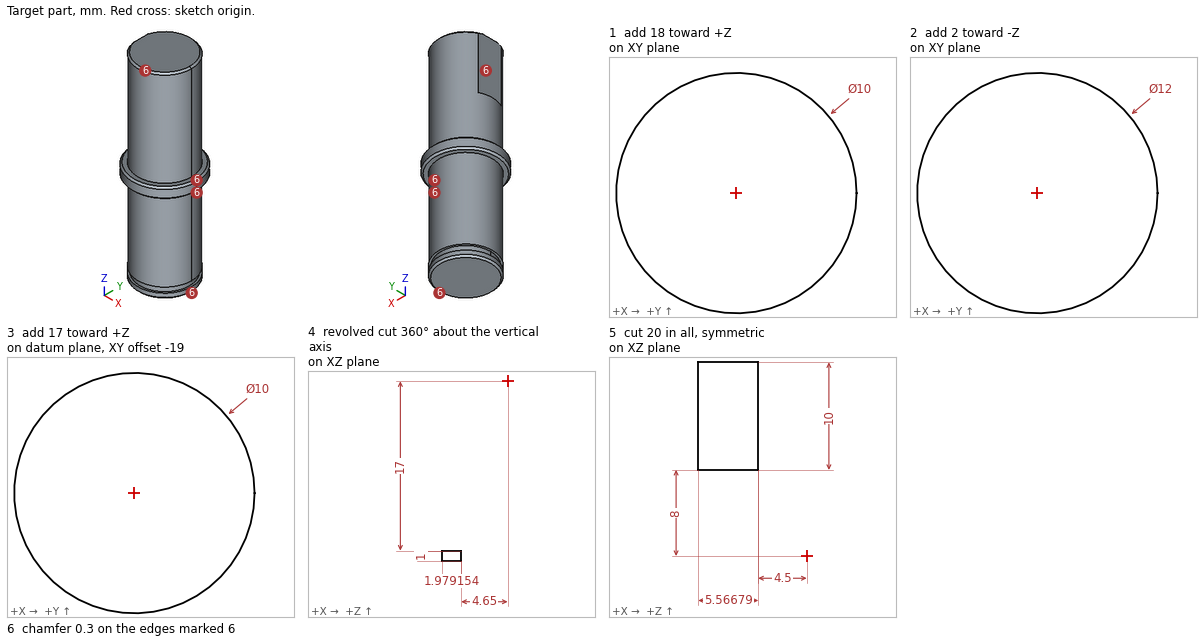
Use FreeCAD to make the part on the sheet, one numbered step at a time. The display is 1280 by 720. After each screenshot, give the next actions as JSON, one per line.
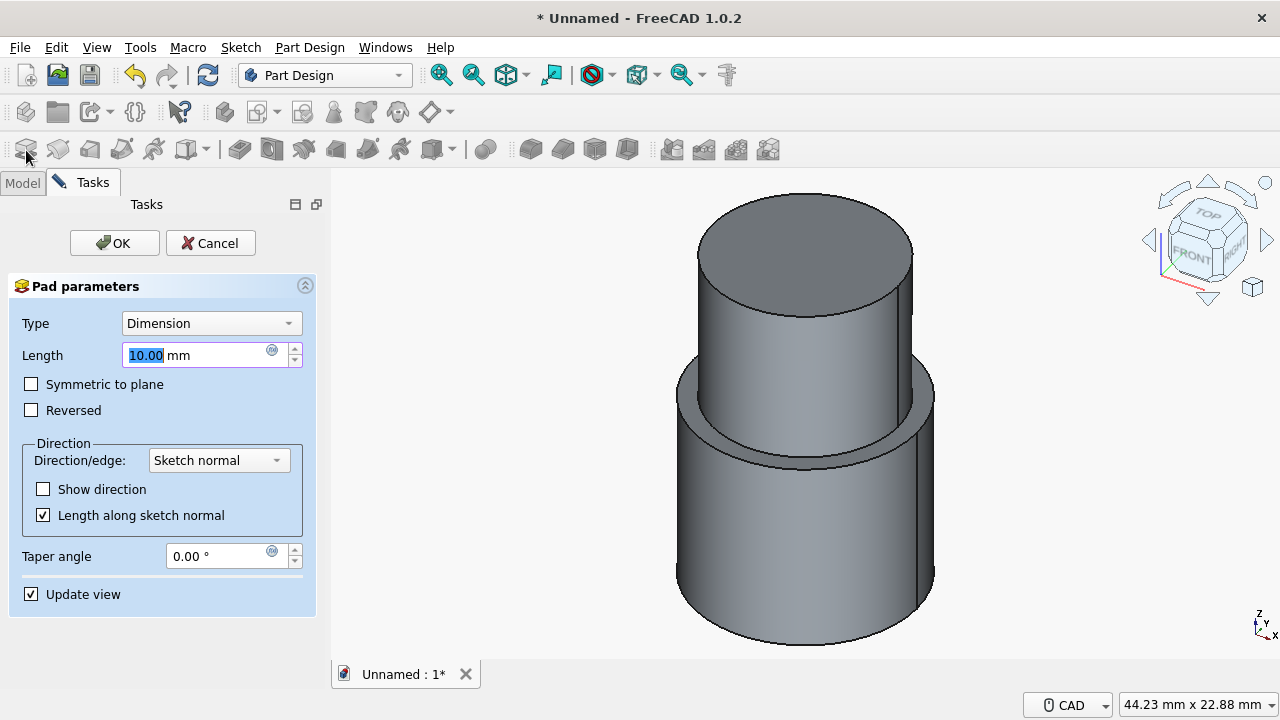
{"action": "type", "text": "2"}
{"action": "key", "text": "Tab"}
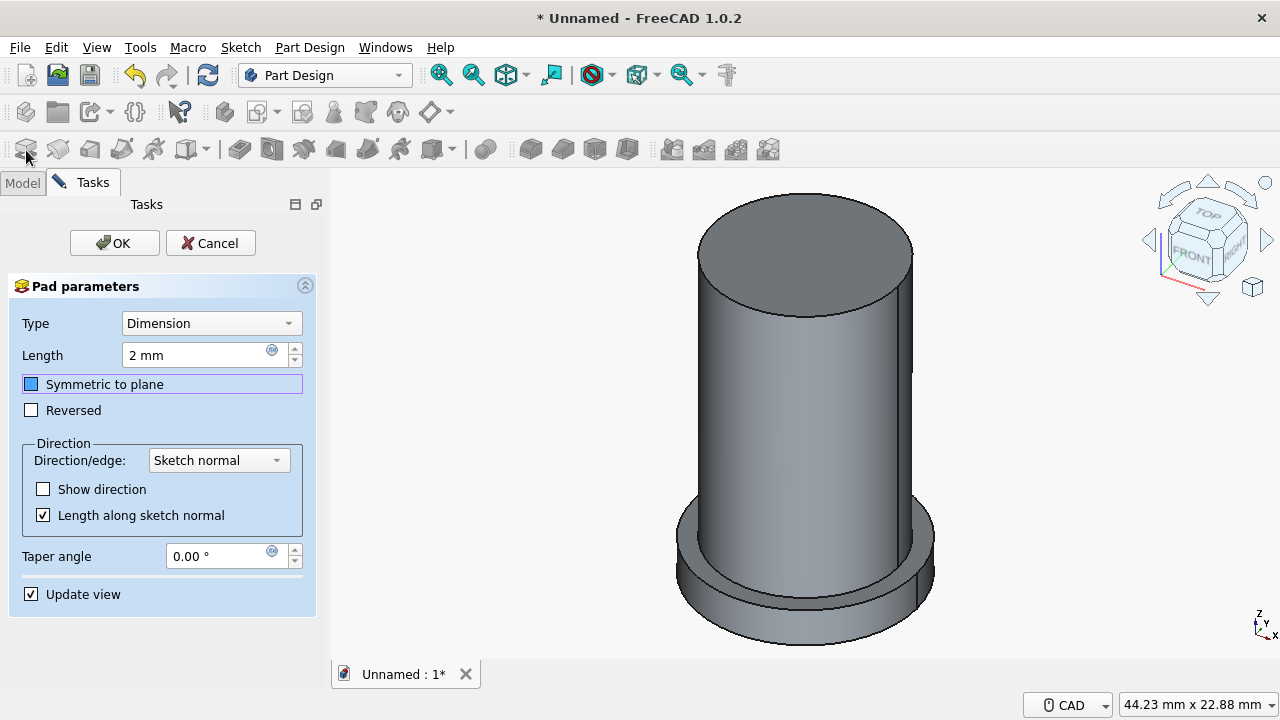
{"action": "left_click", "coordinate": [30, 410]}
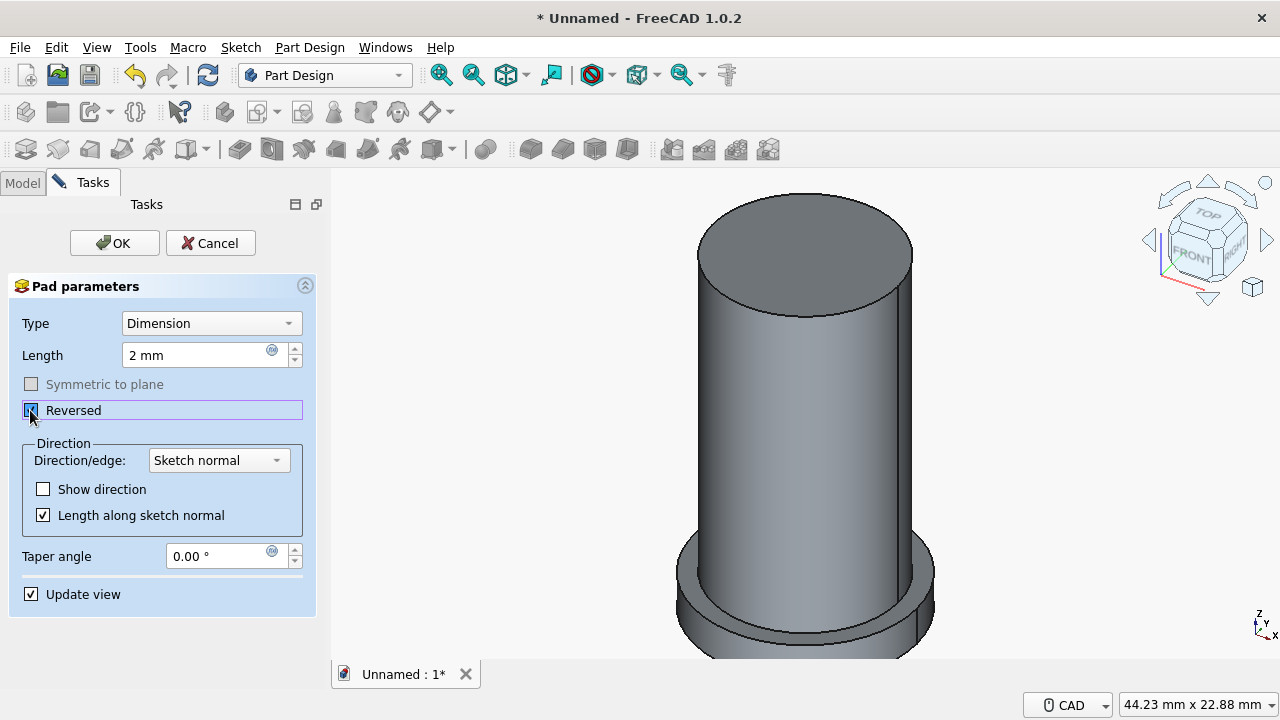
{"action": "left_click", "coordinate": [115, 243]}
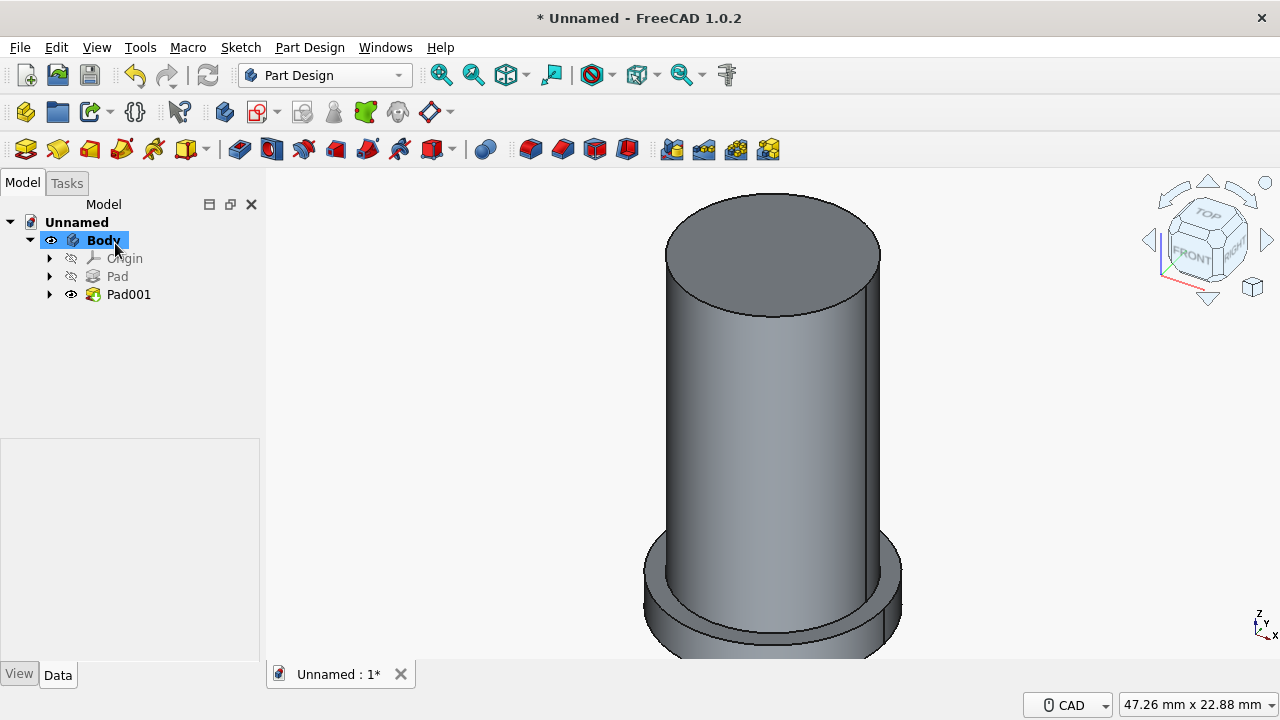
{"action": "left_click", "coordinate": [442, 76]}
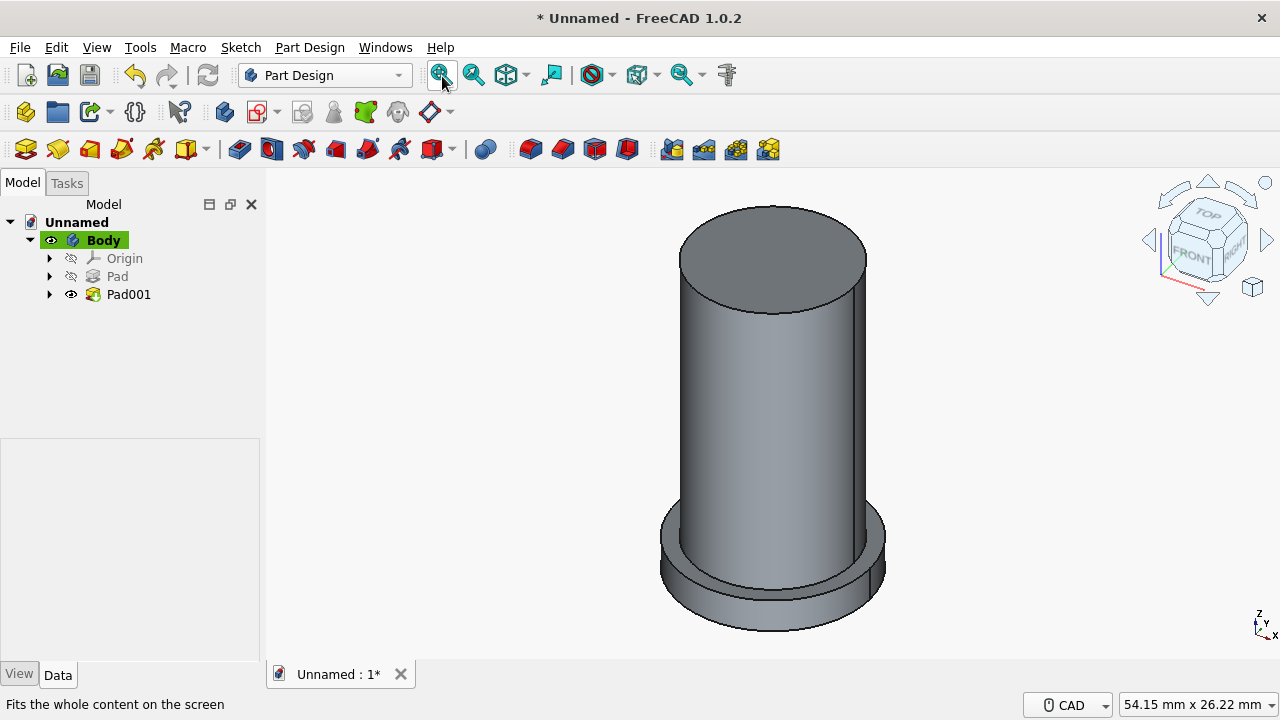
{"action": "left_click", "coordinate": [50, 258]}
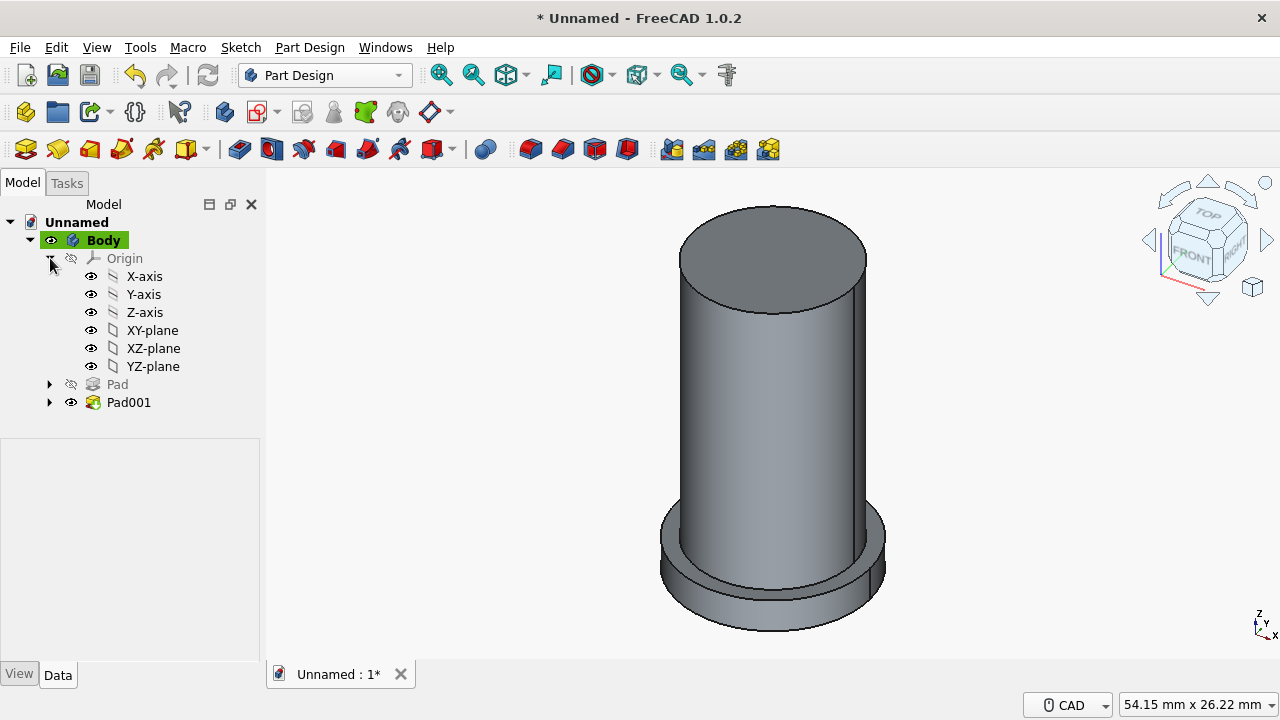
{"action": "left_click", "coordinate": [136, 330]}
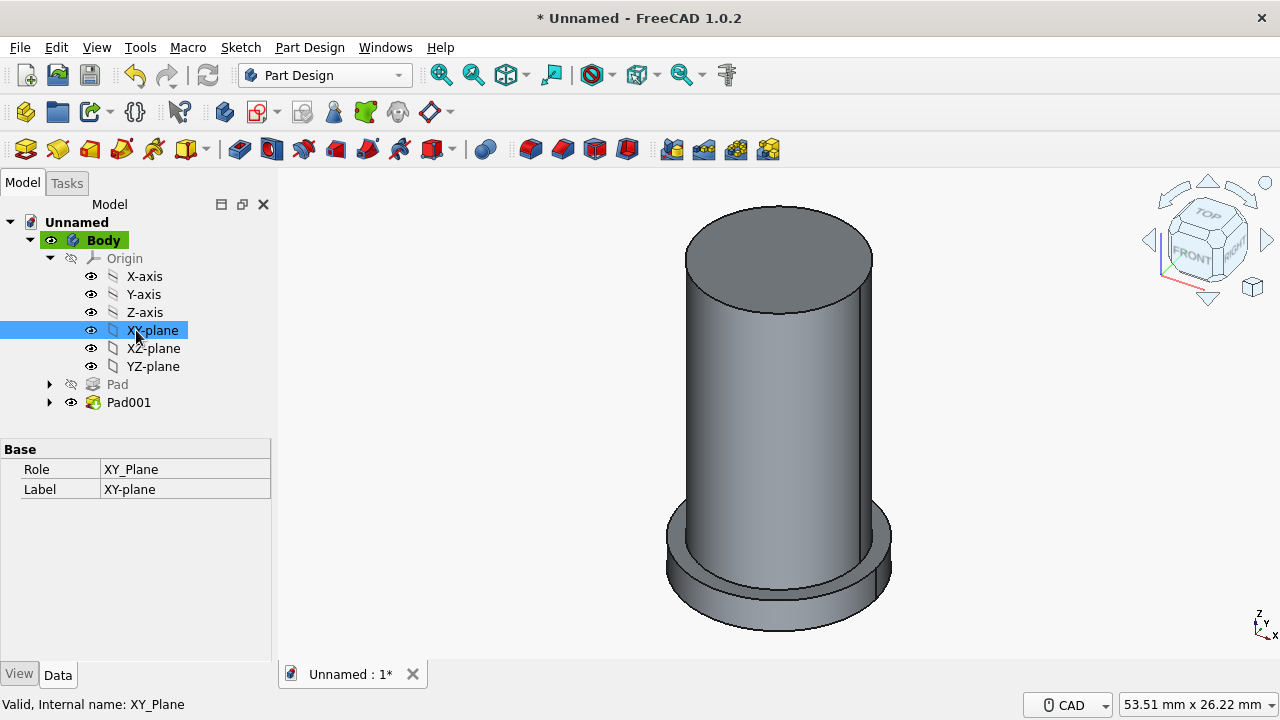
{"action": "left_click", "coordinate": [430, 112]}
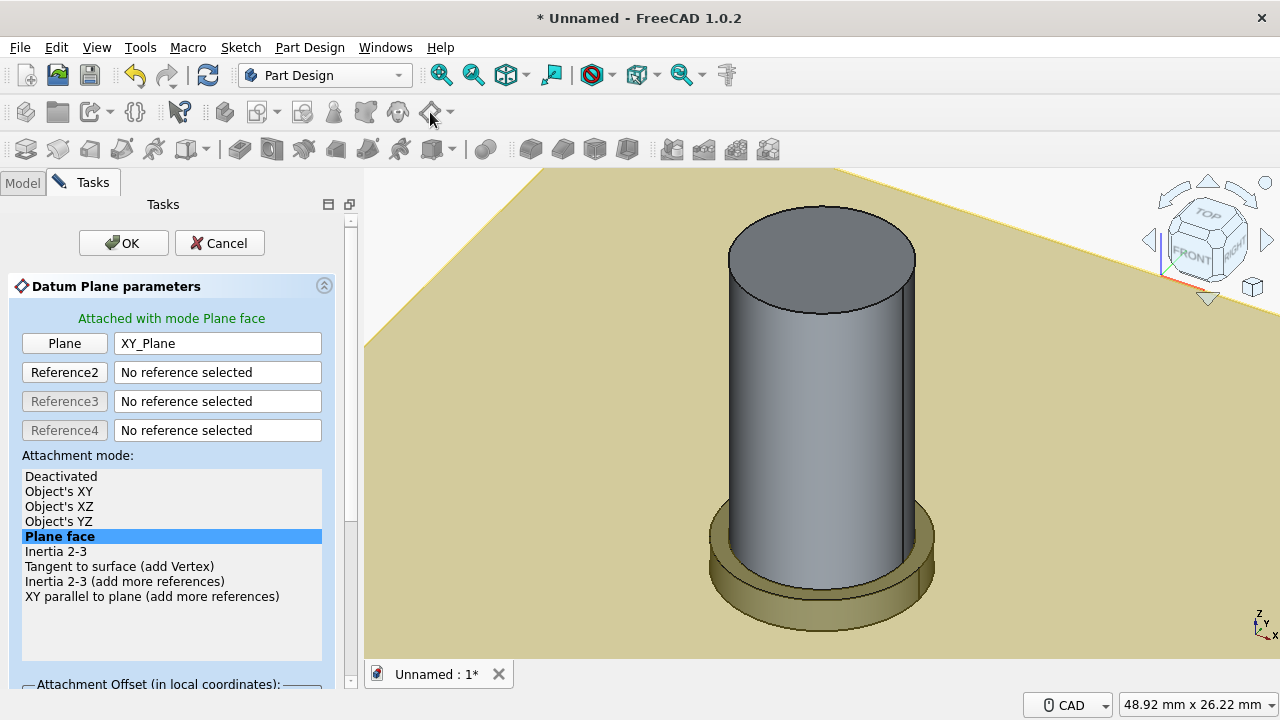
{"action": "scroll", "coordinate": [351, 451], "scroll_direction": "down", "scroll_amount": 3}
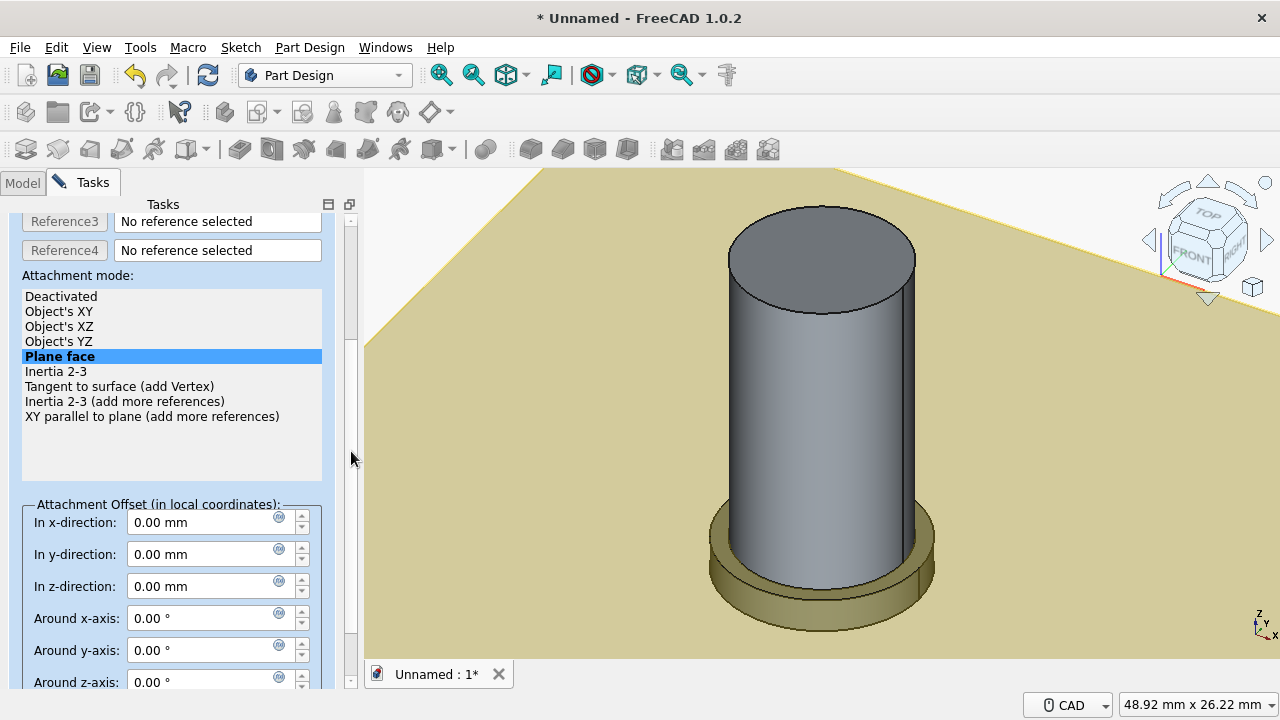
{"action": "triple_click", "coordinate": [210, 586]}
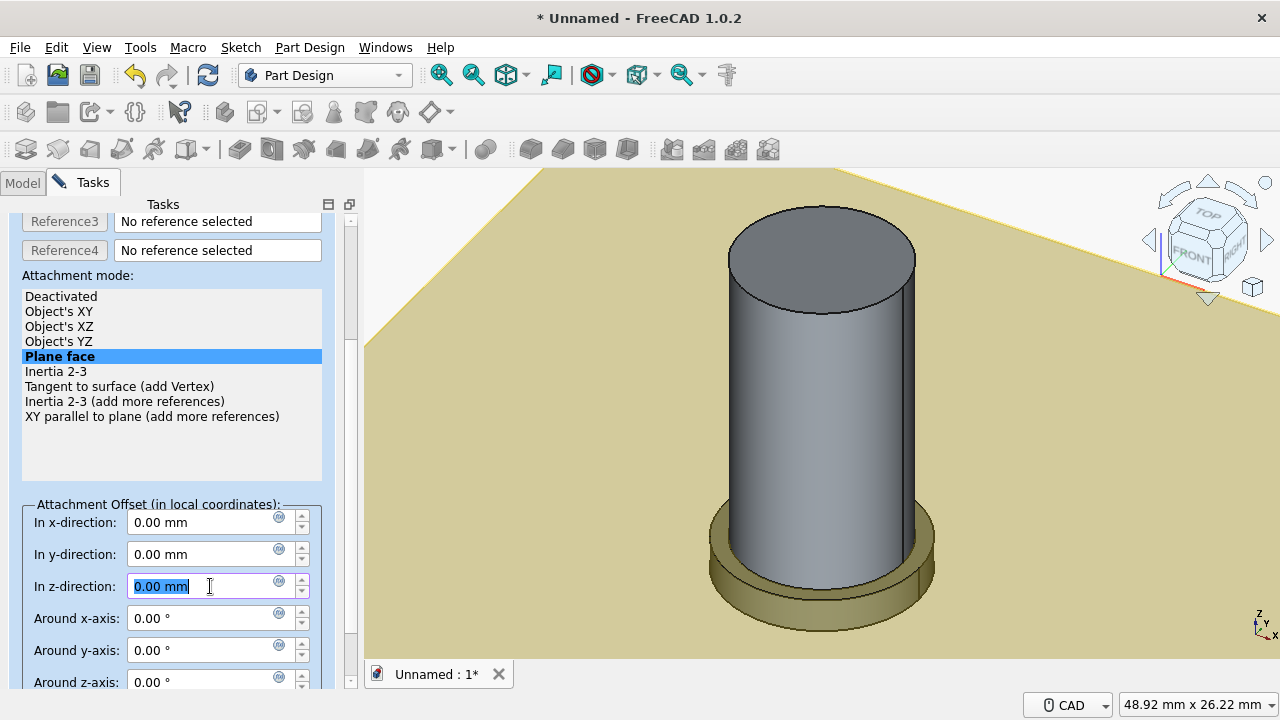
{"action": "type", "text": "-19"}
{"action": "key", "text": "Tab"}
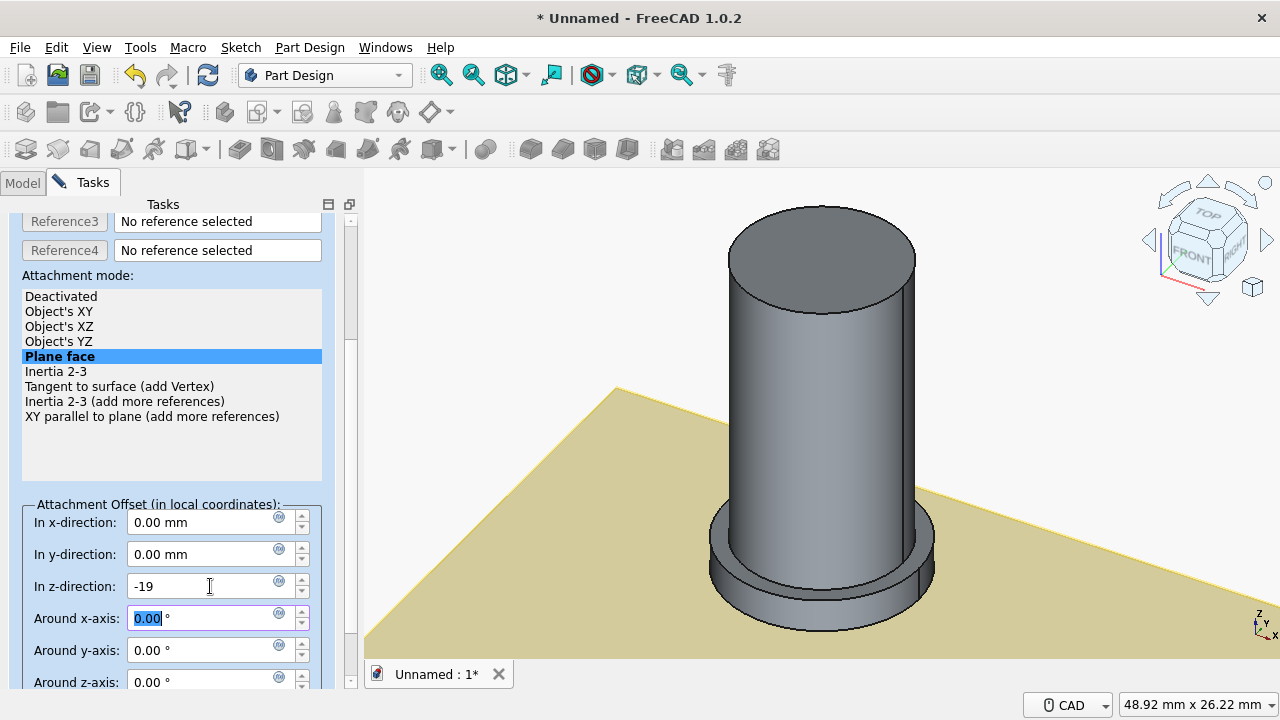
{"action": "scroll", "coordinate": [351, 451], "scroll_direction": "up", "scroll_amount": 4}